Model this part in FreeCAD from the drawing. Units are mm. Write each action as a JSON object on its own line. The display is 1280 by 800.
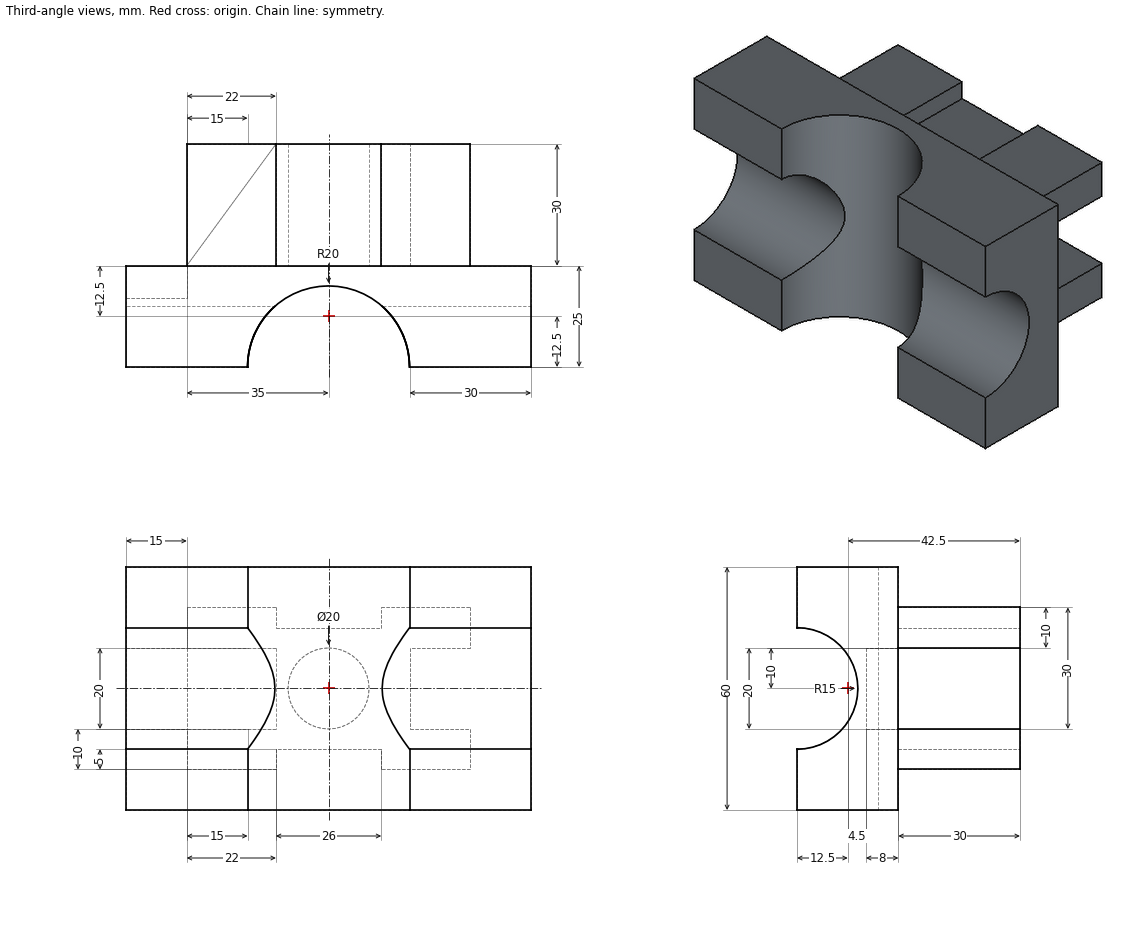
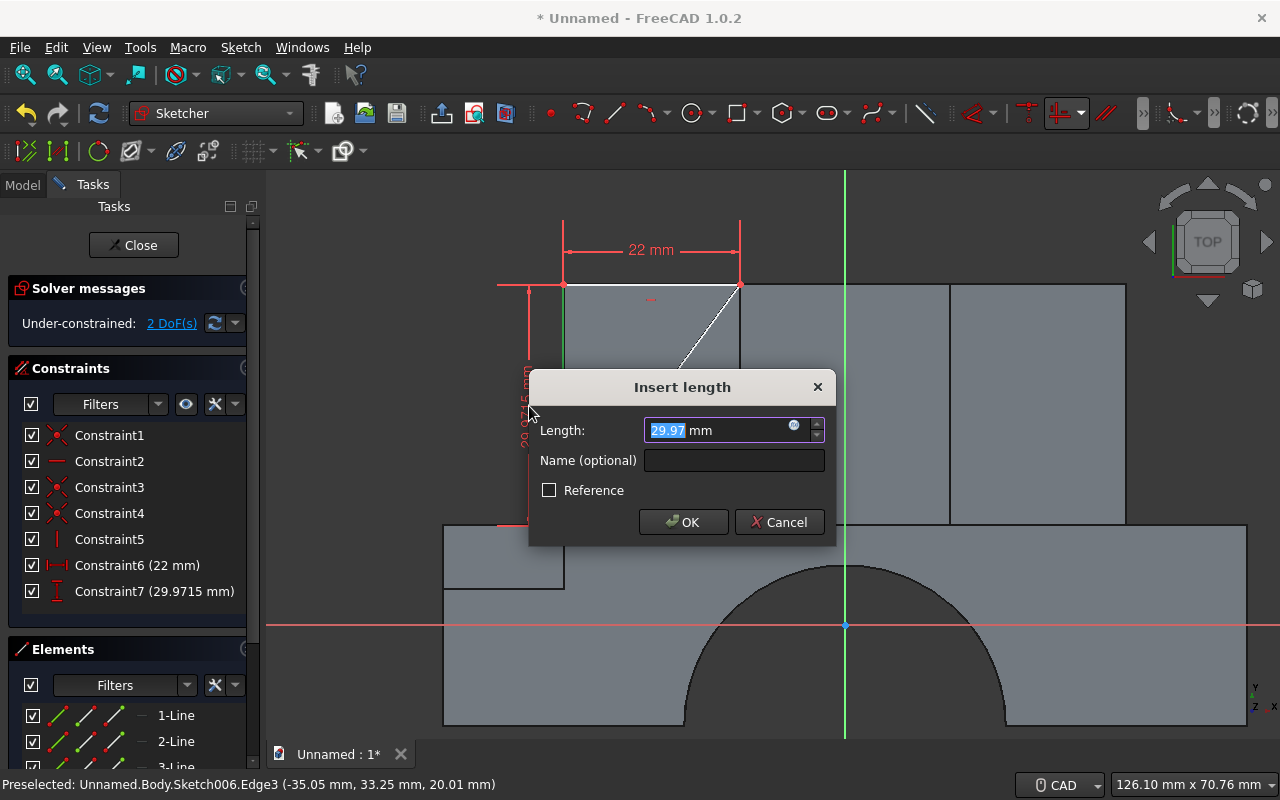
{"action": "type", "text": "30"}
{"action": "key", "text": "Return"}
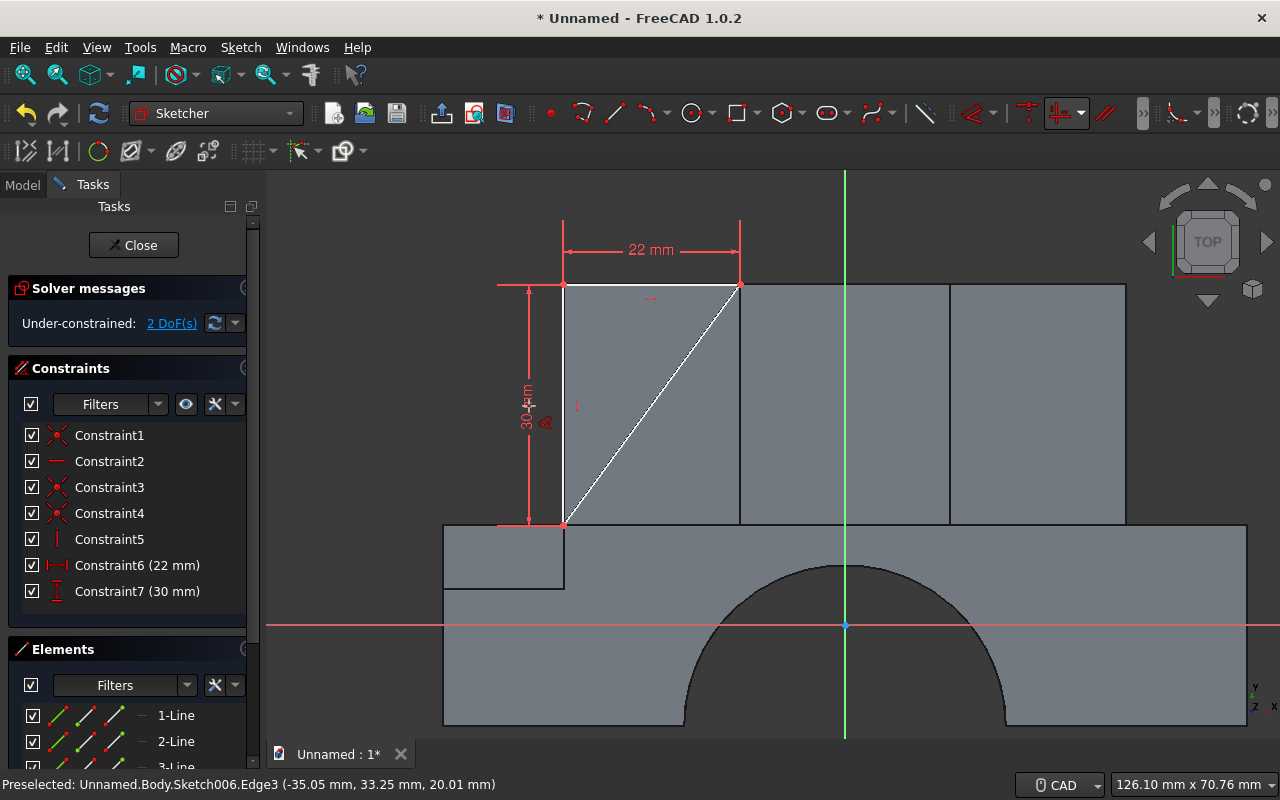
{"action": "left_click", "coordinate": [563, 526]}
{"action": "left_click", "coordinate": [704, 659]}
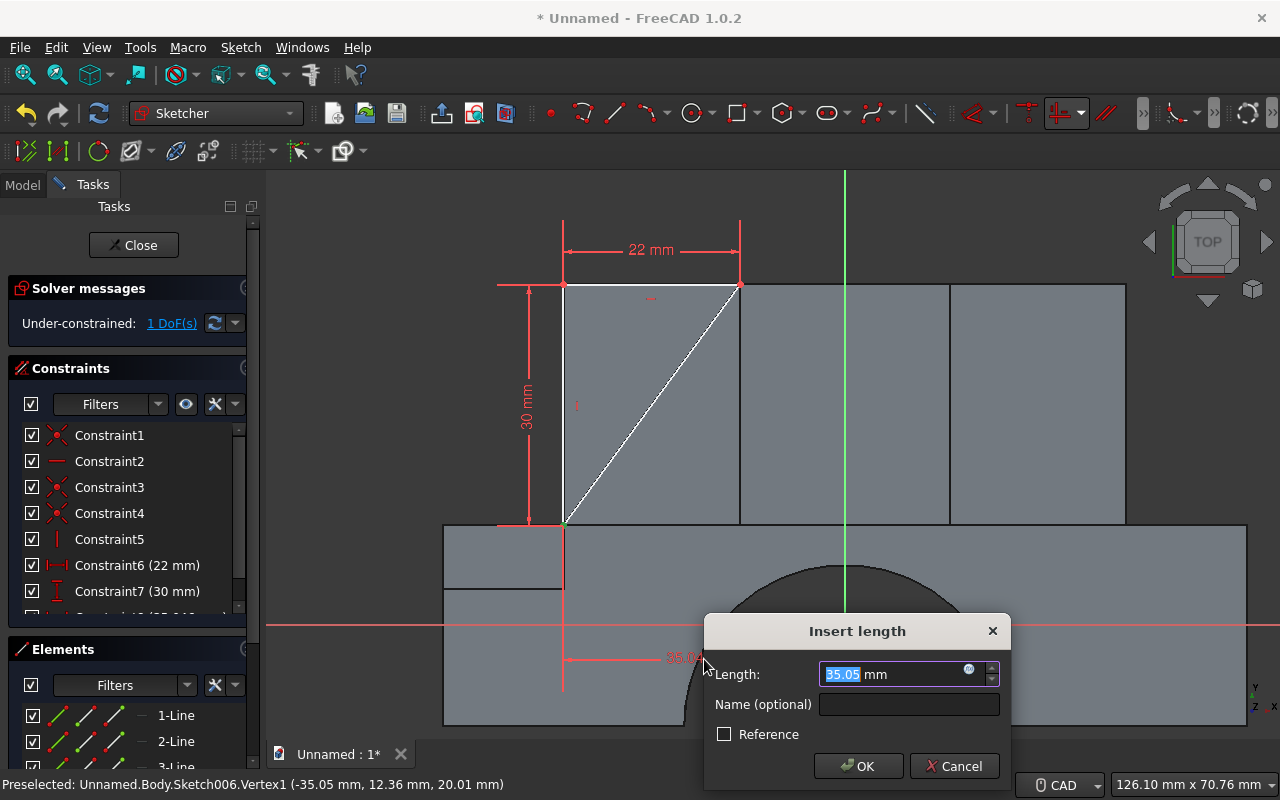
{"action": "type", "text": "35"}
{"action": "key", "text": "Return"}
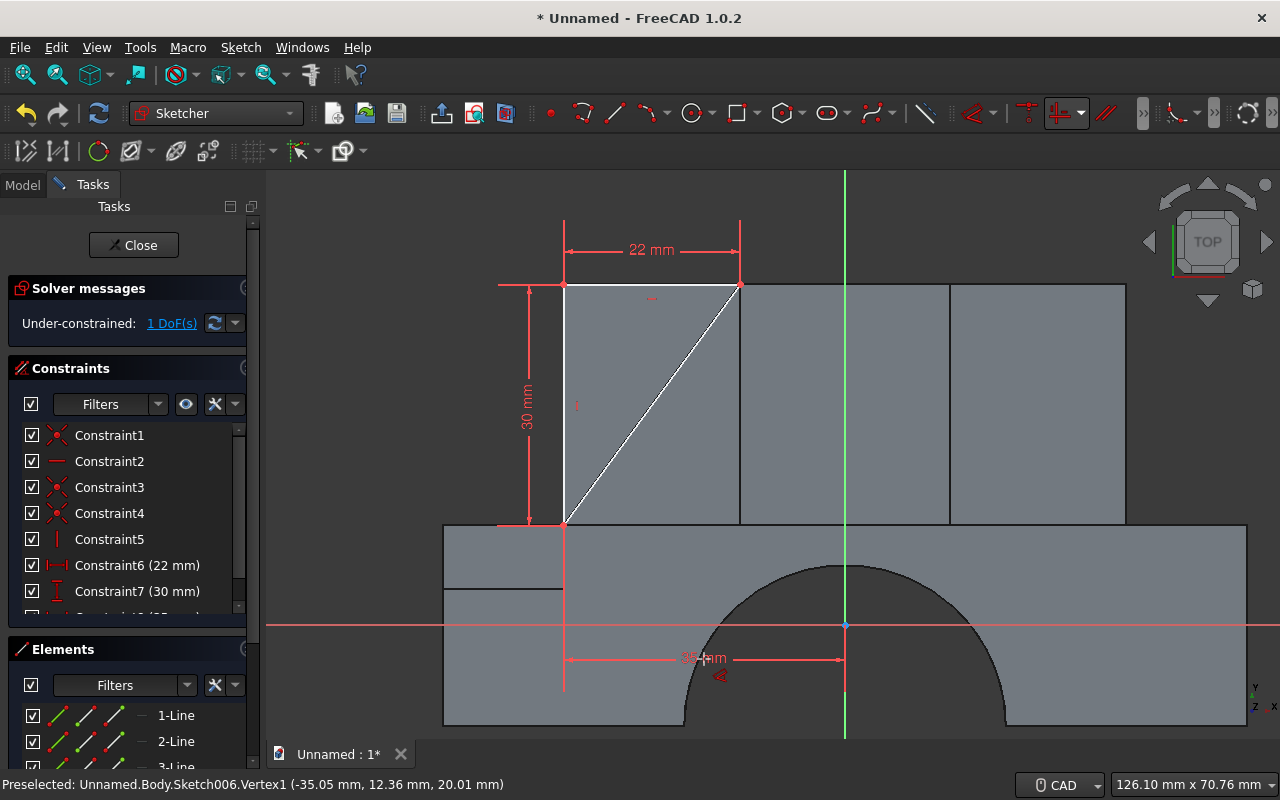
{"action": "left_click", "coordinate": [564, 526]}
{"action": "left_click", "coordinate": [879, 576]}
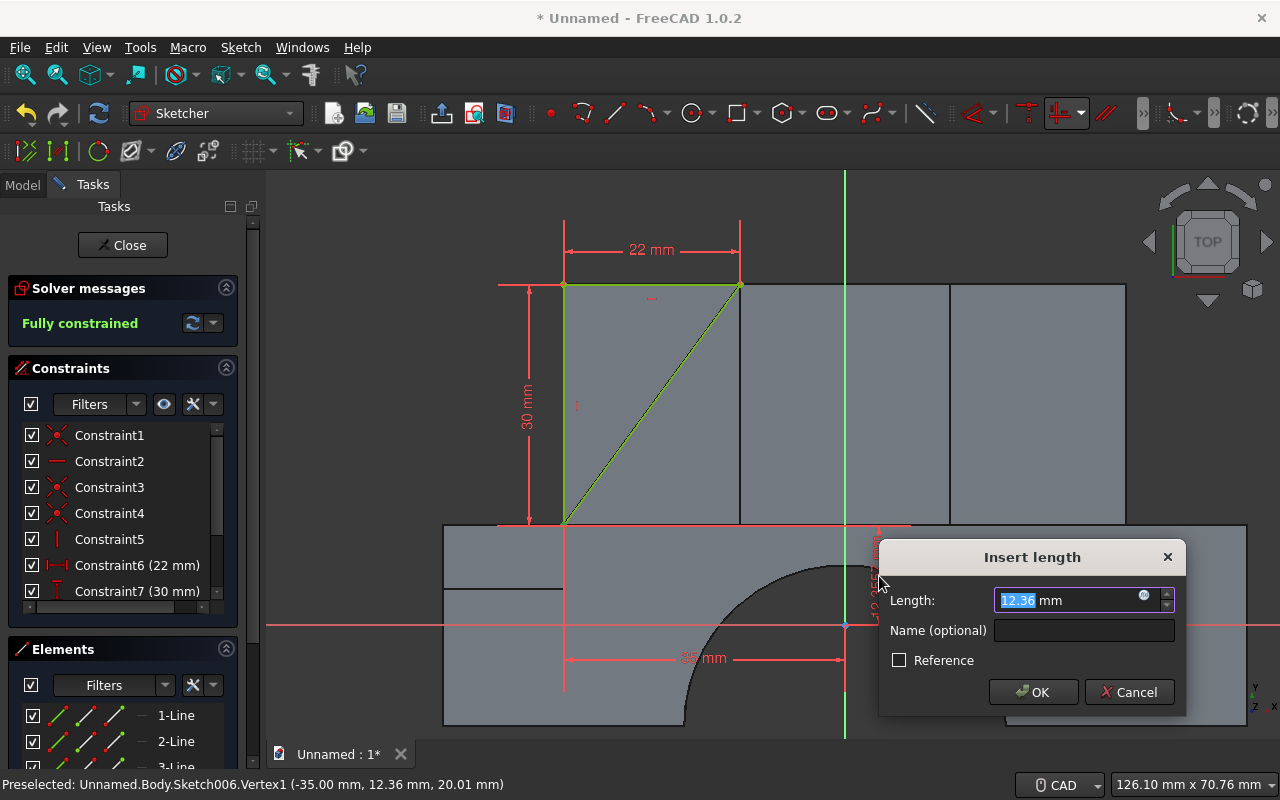
{"action": "type", "text": "12.5"}
{"action": "key", "text": "Return"}
{"action": "key", "text": "Escape"}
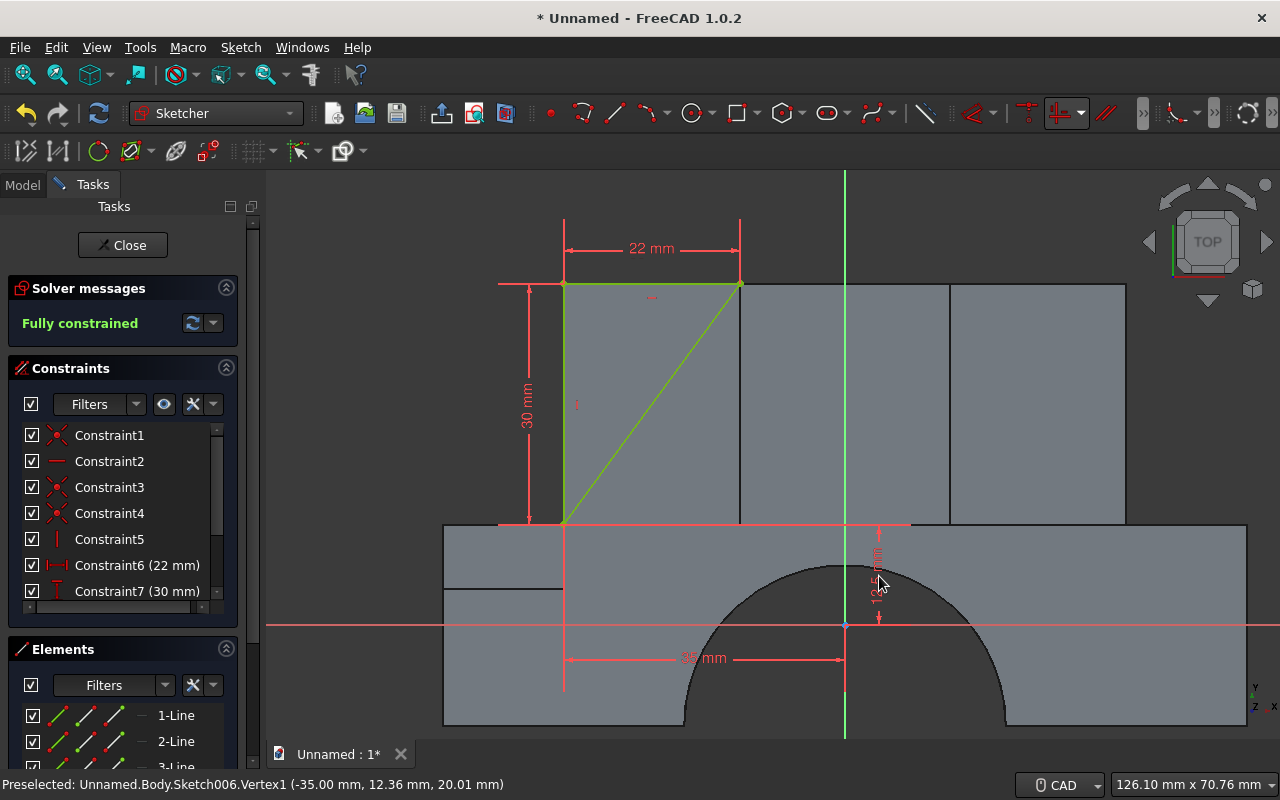
{"action": "left_click", "coordinate": [123, 245]}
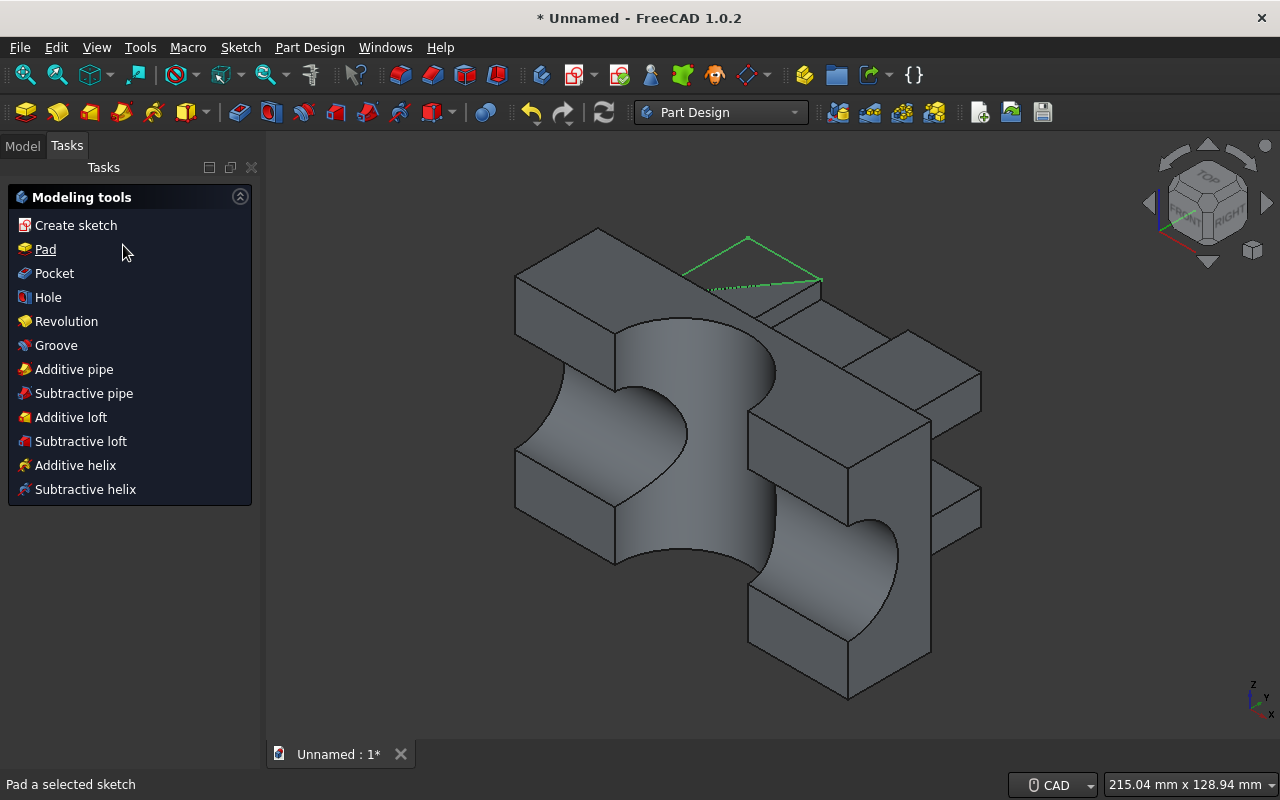
{"action": "left_click", "coordinate": [26, 112]}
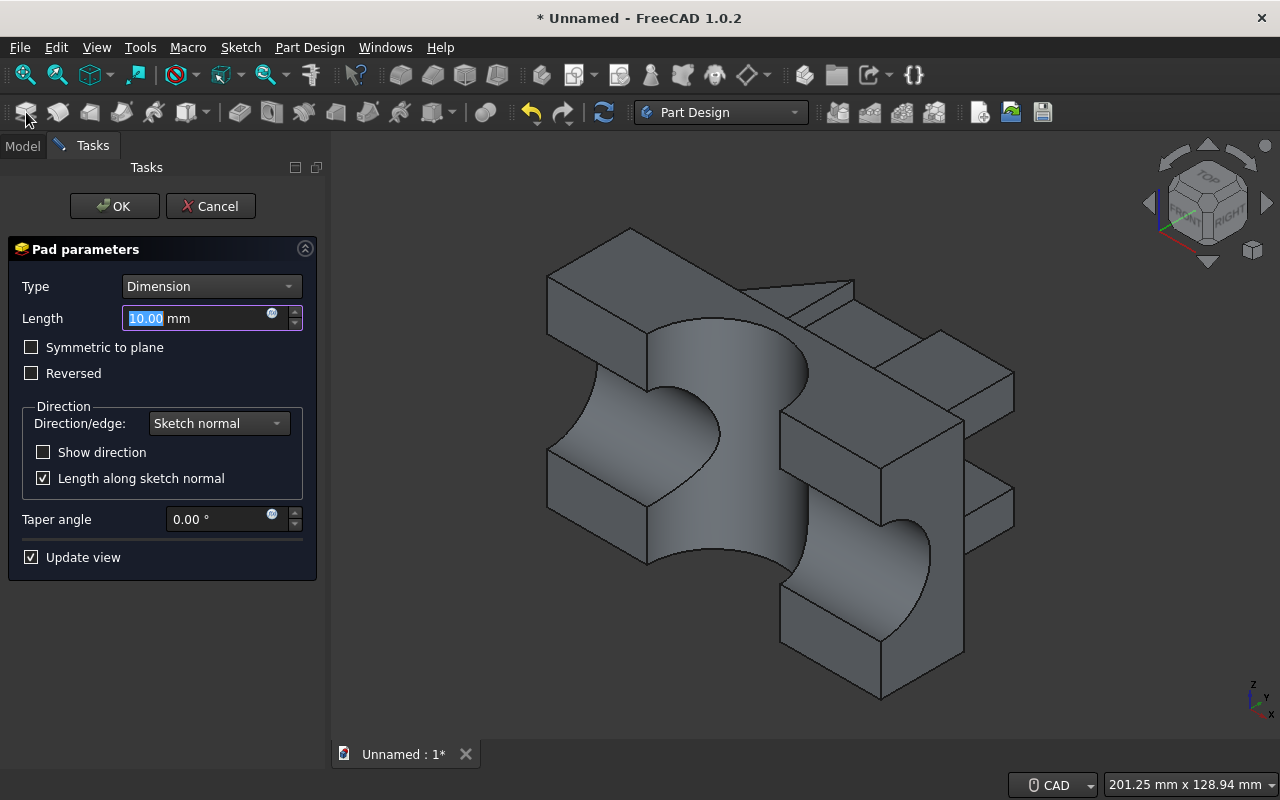
{"action": "type", "text": "10"}
{"action": "key", "text": "Tab"}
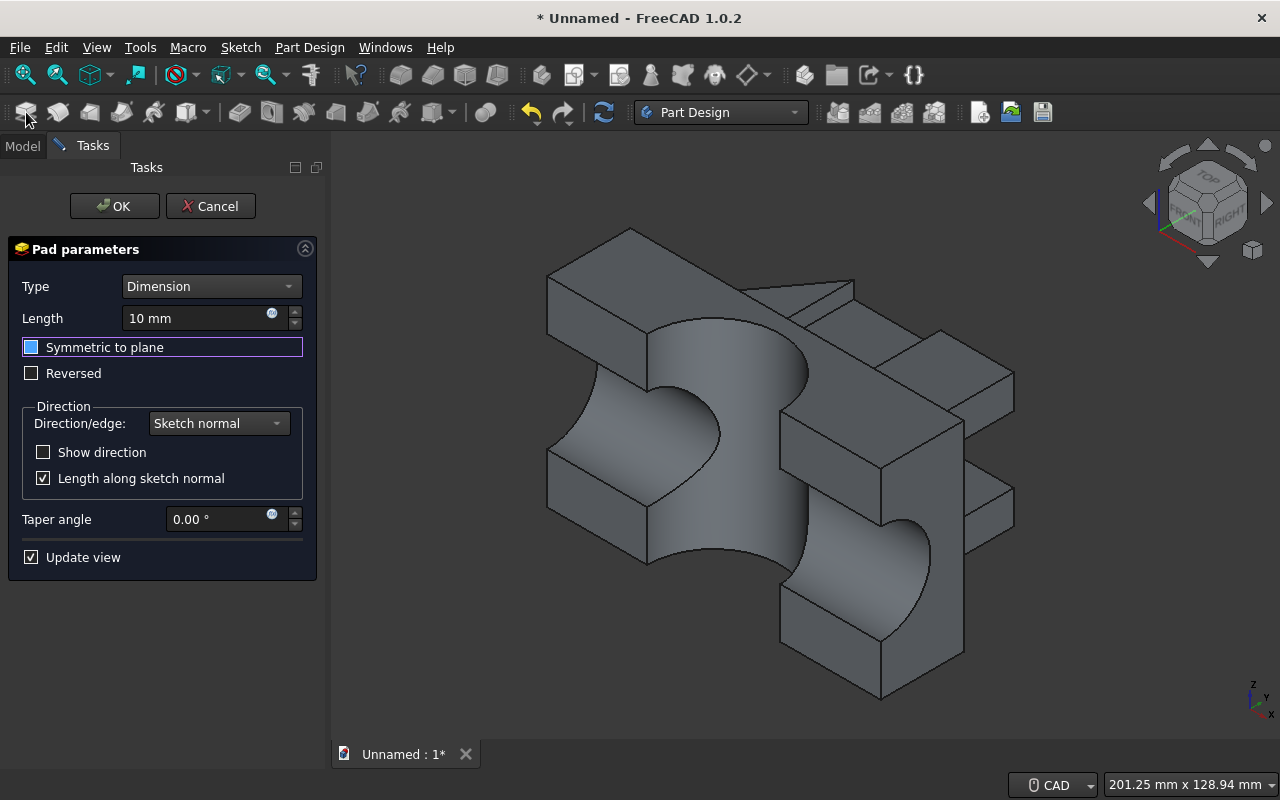
{"action": "left_click", "coordinate": [30, 373]}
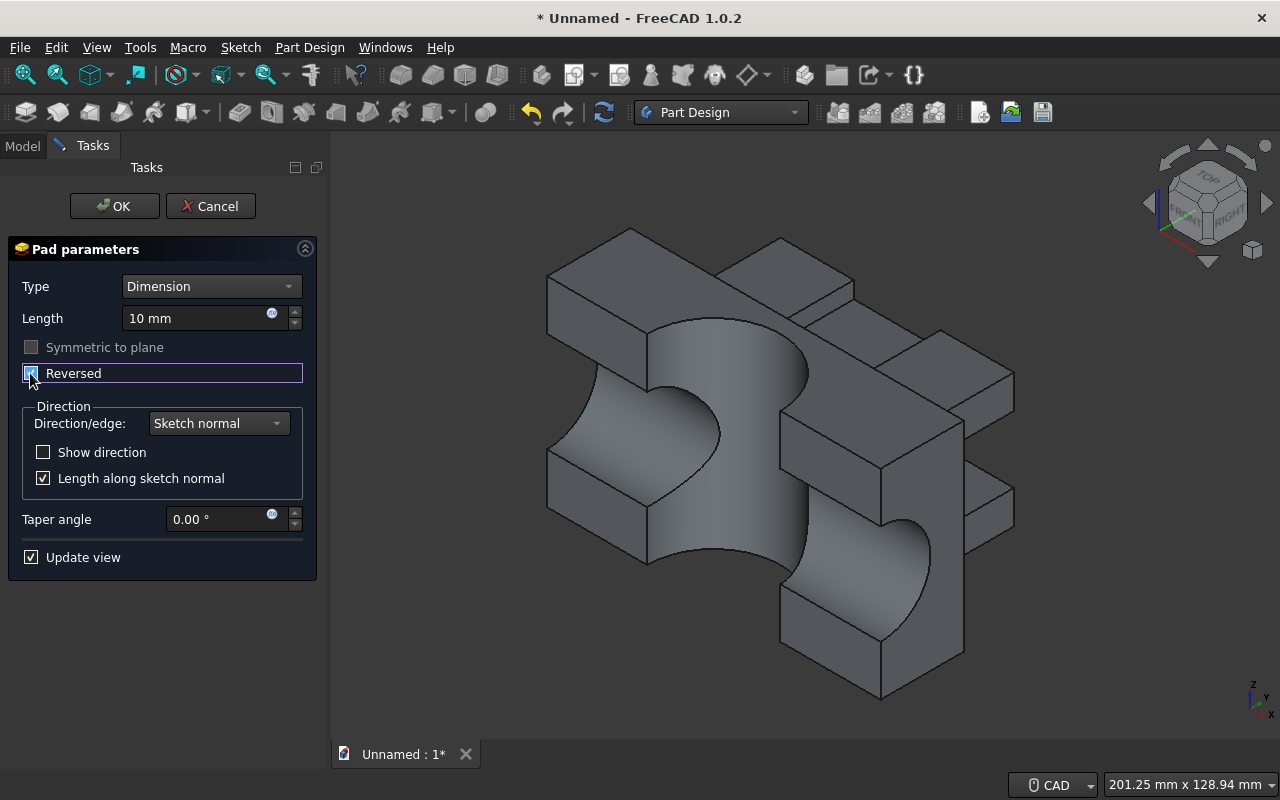
{"action": "left_click", "coordinate": [115, 206]}